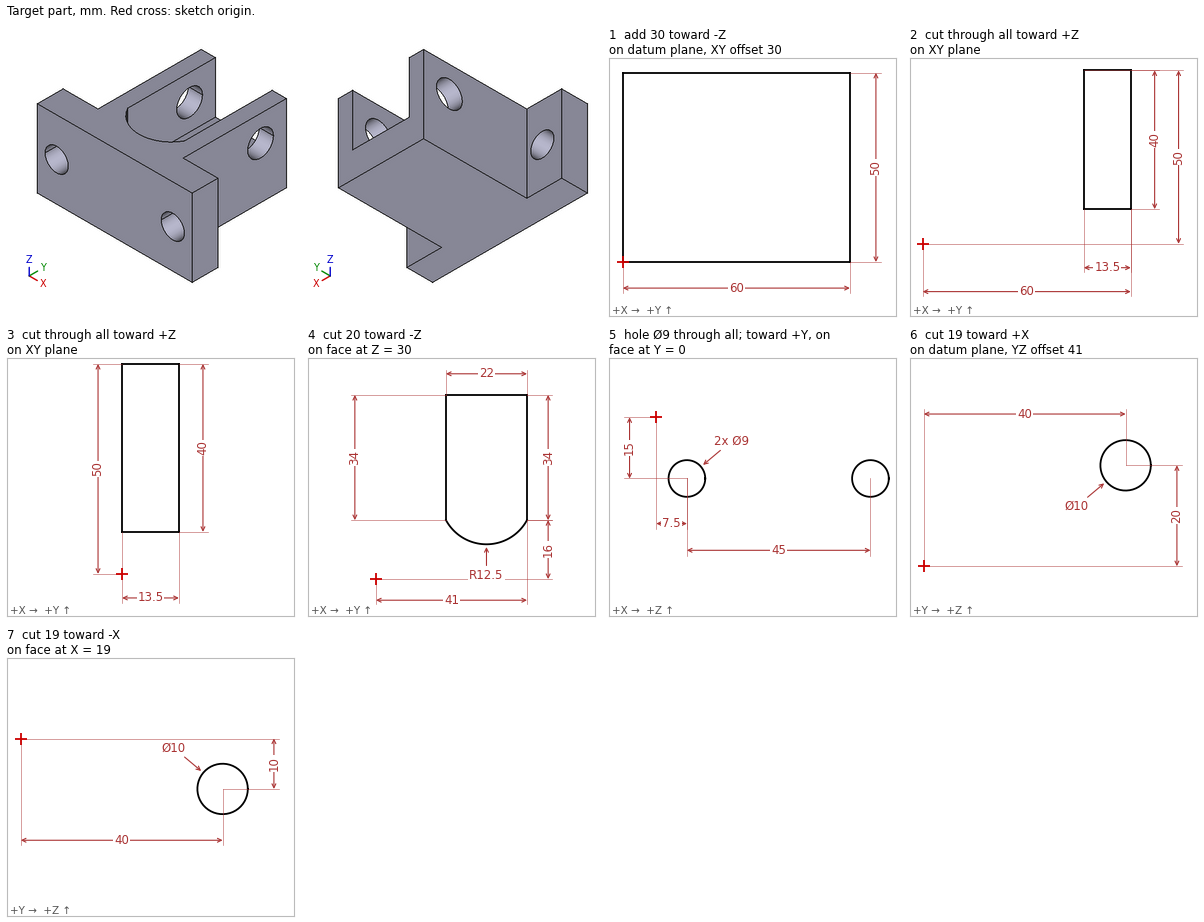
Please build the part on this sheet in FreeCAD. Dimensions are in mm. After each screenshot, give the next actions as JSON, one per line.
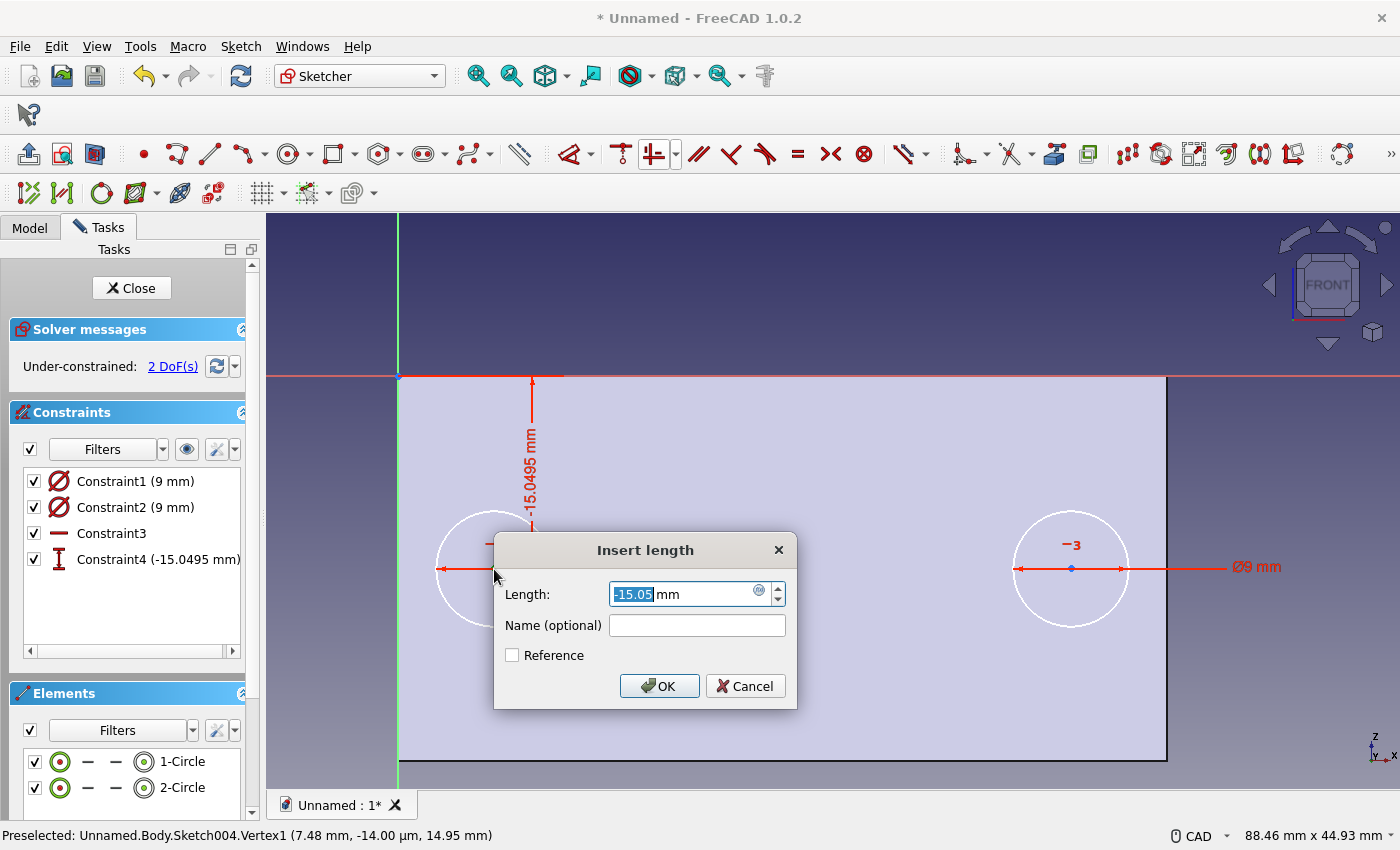
{"action": "type", "text": "-15"}
{"action": "key", "text": "Return"}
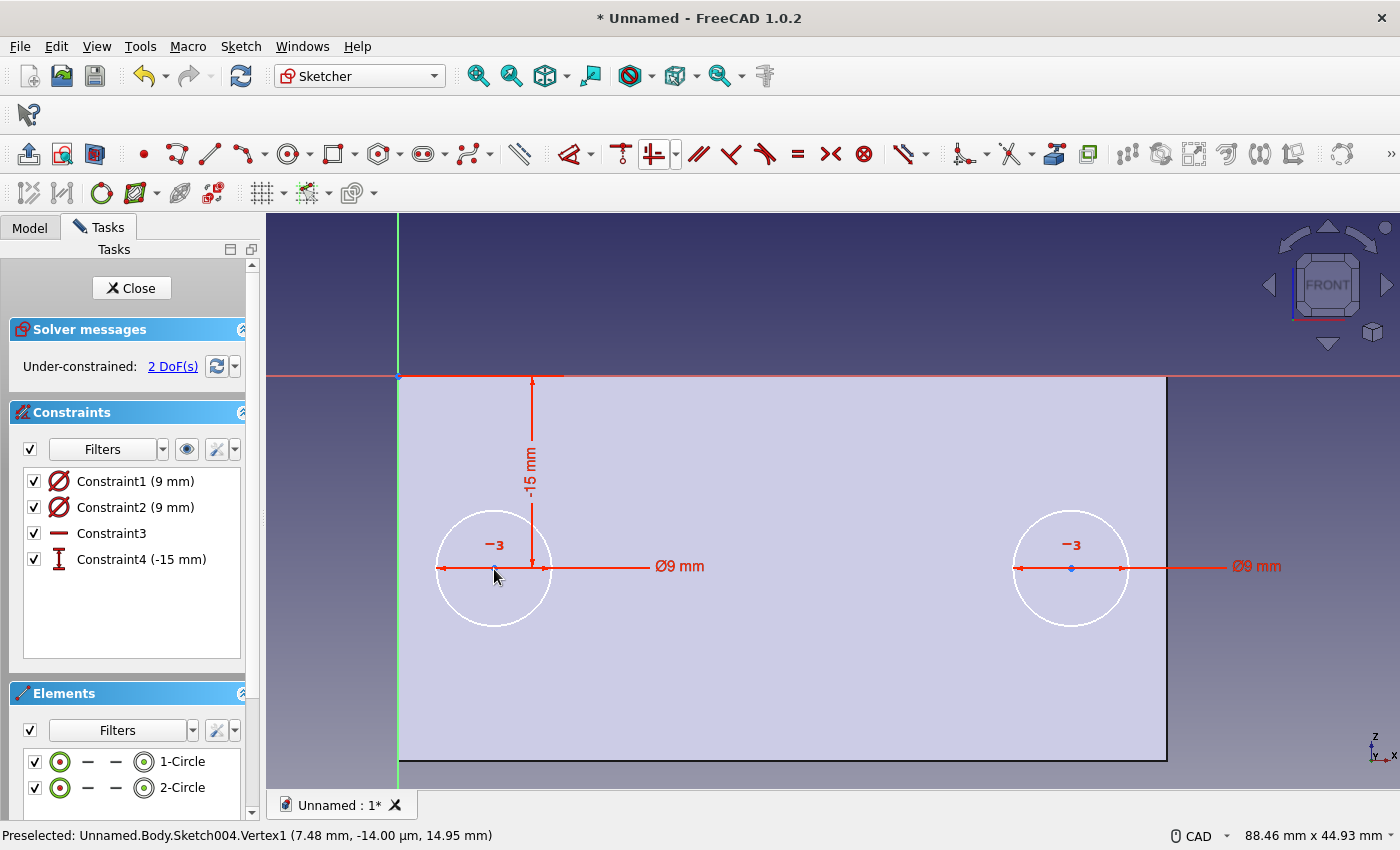
{"action": "left_click", "coordinate": [494, 568]}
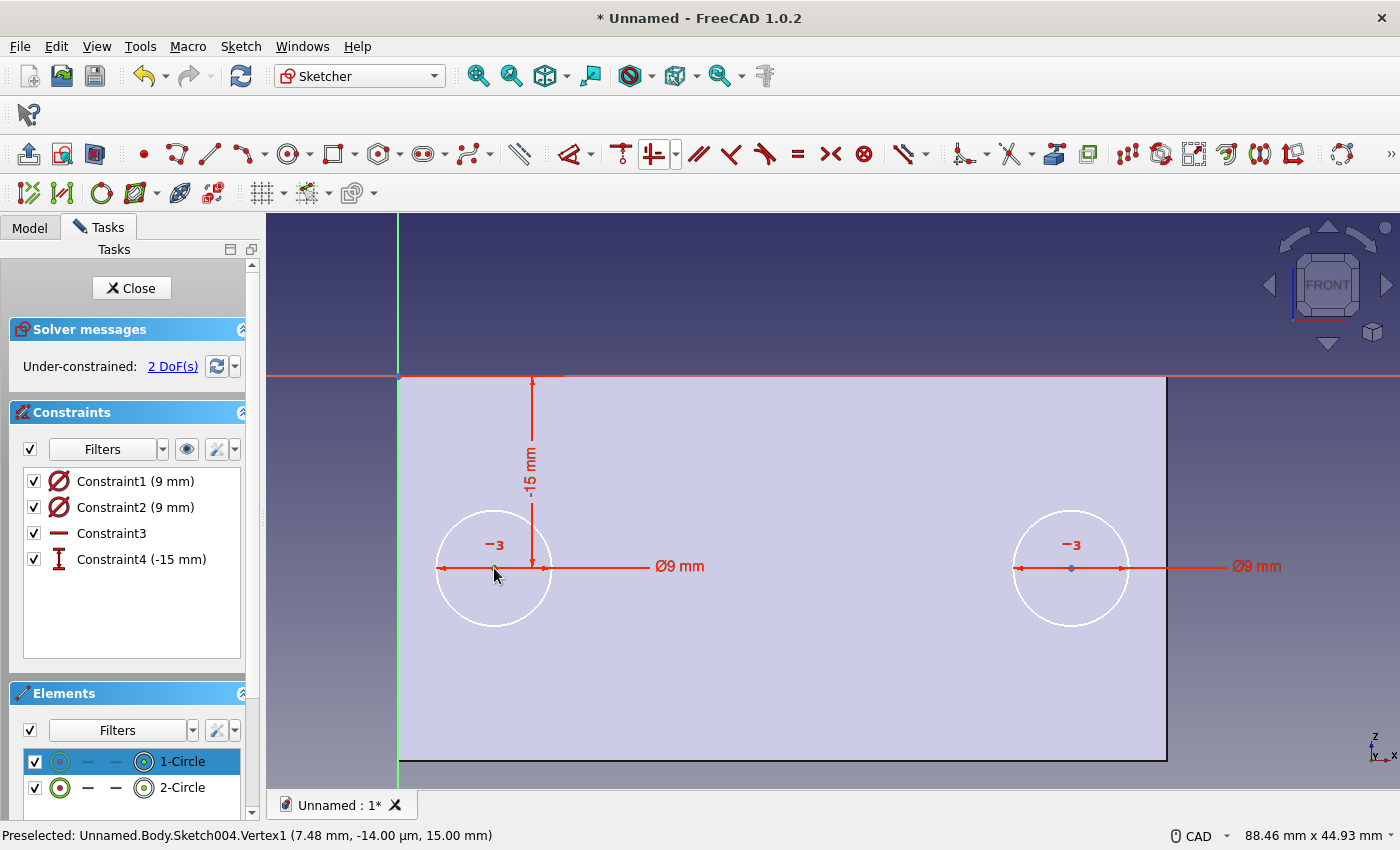
{"action": "key", "text": "l"}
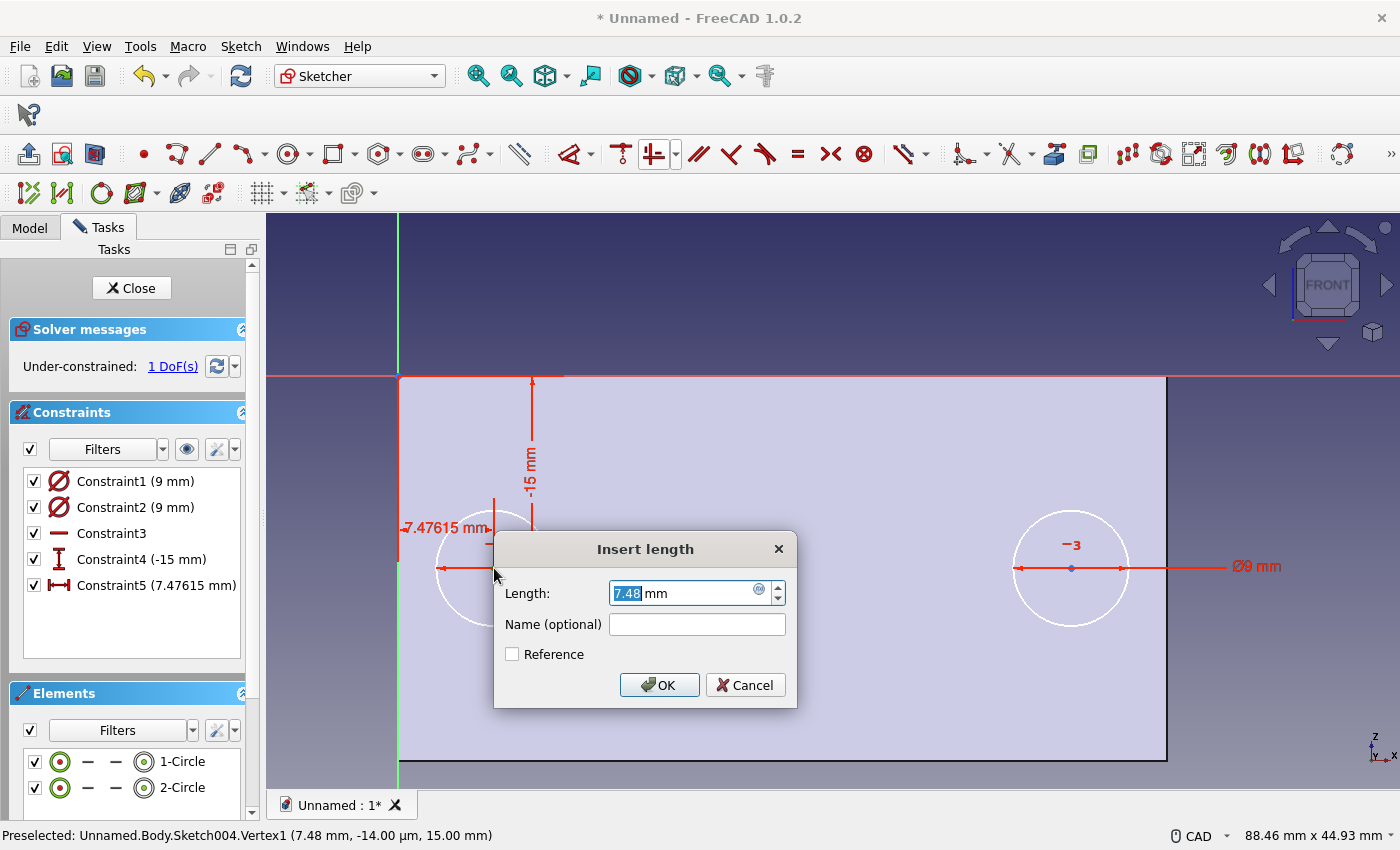
{"action": "type", "text": "7.5"}
{"action": "key", "text": "Return"}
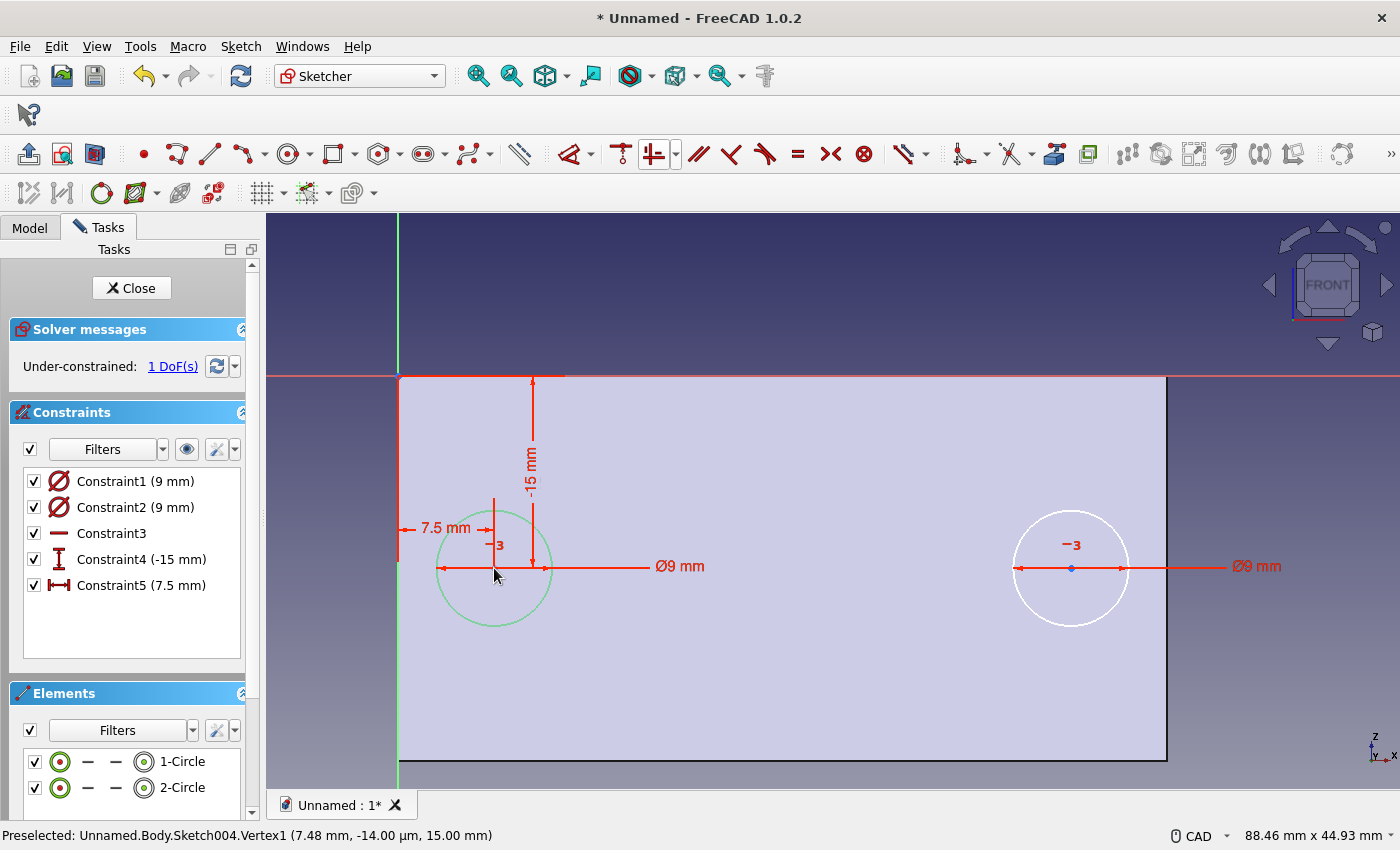
{"action": "left_click", "coordinate": [494, 568]}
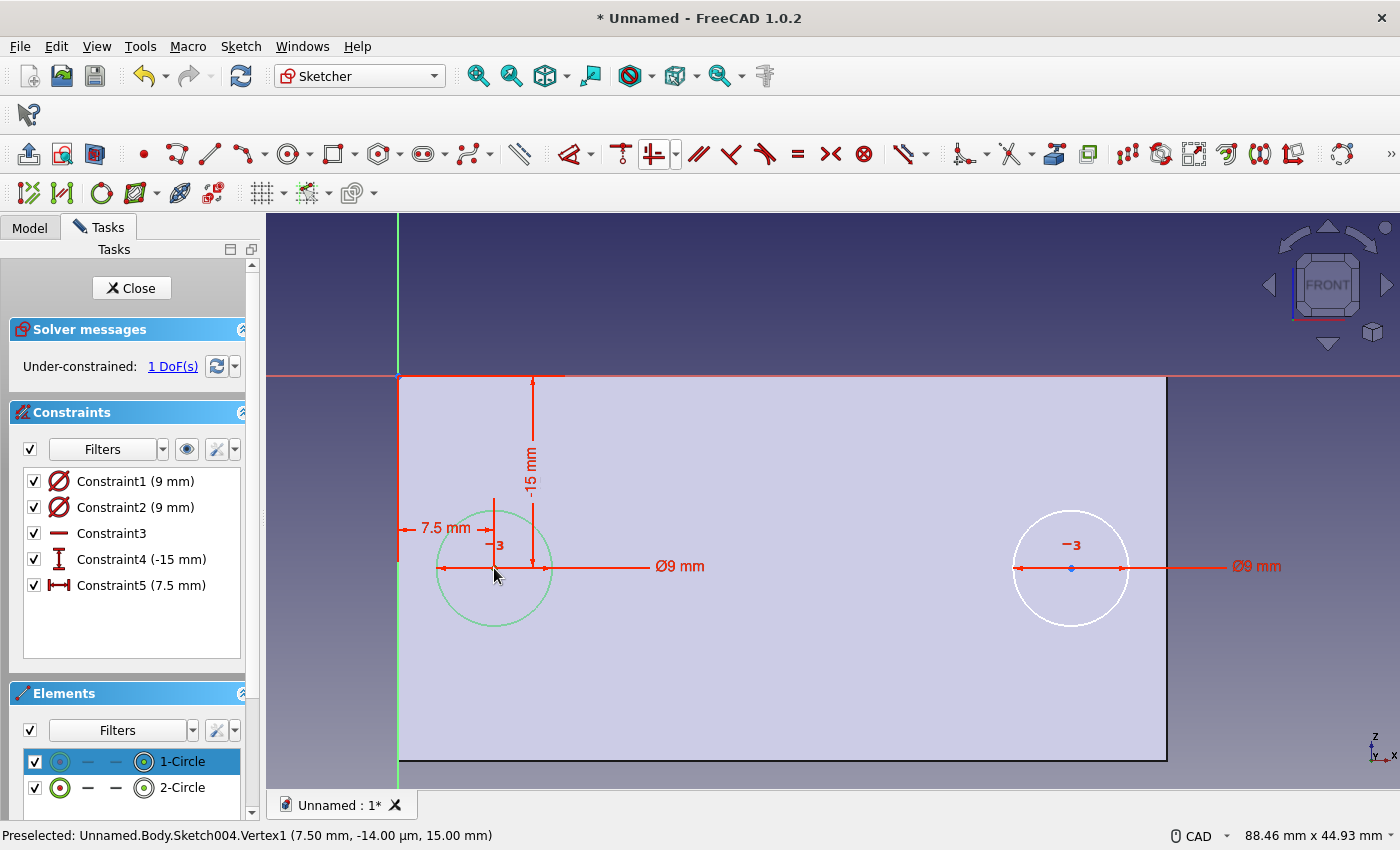
{"action": "left_click", "coordinate": [1071, 568]}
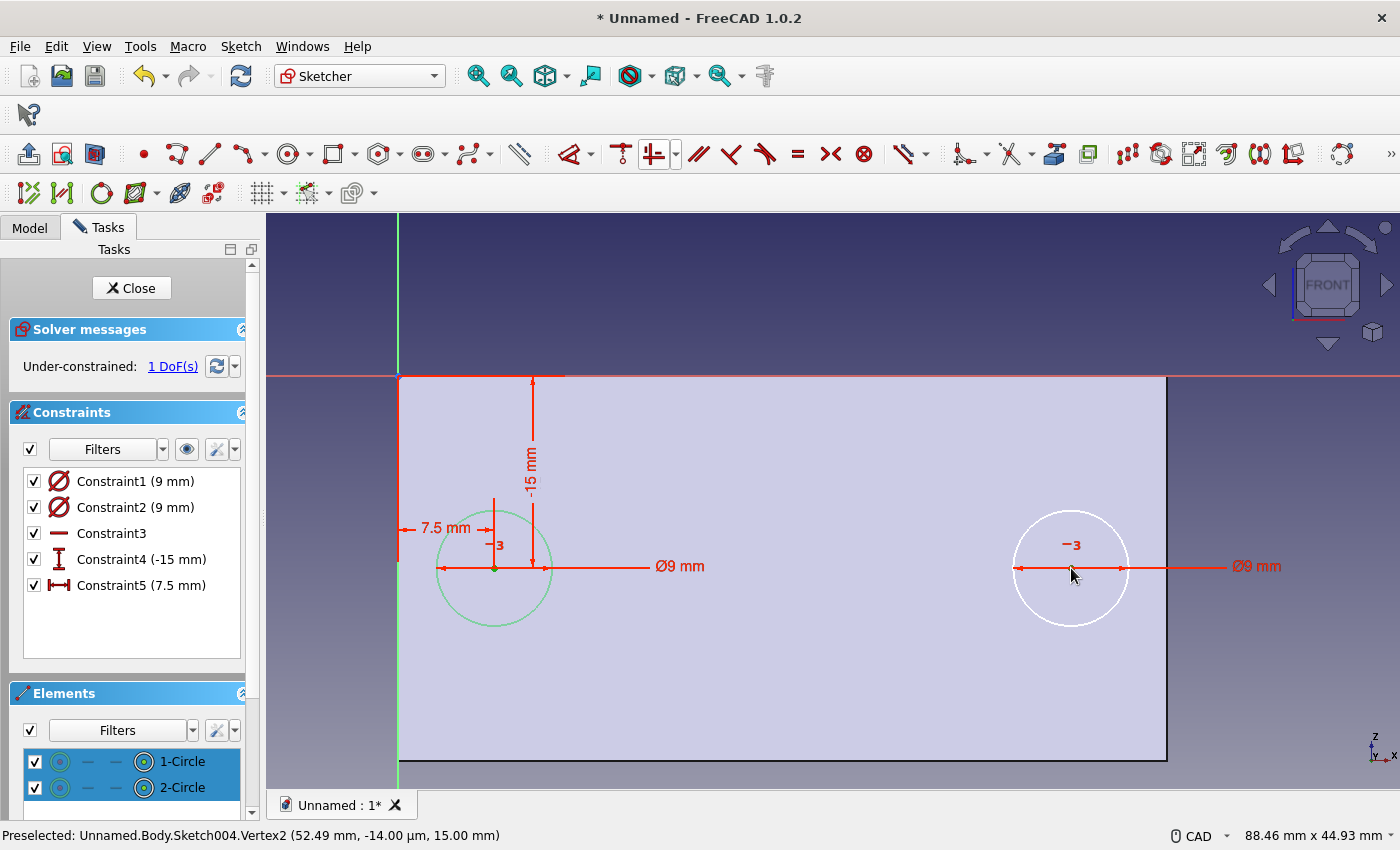
{"action": "key", "text": "l"}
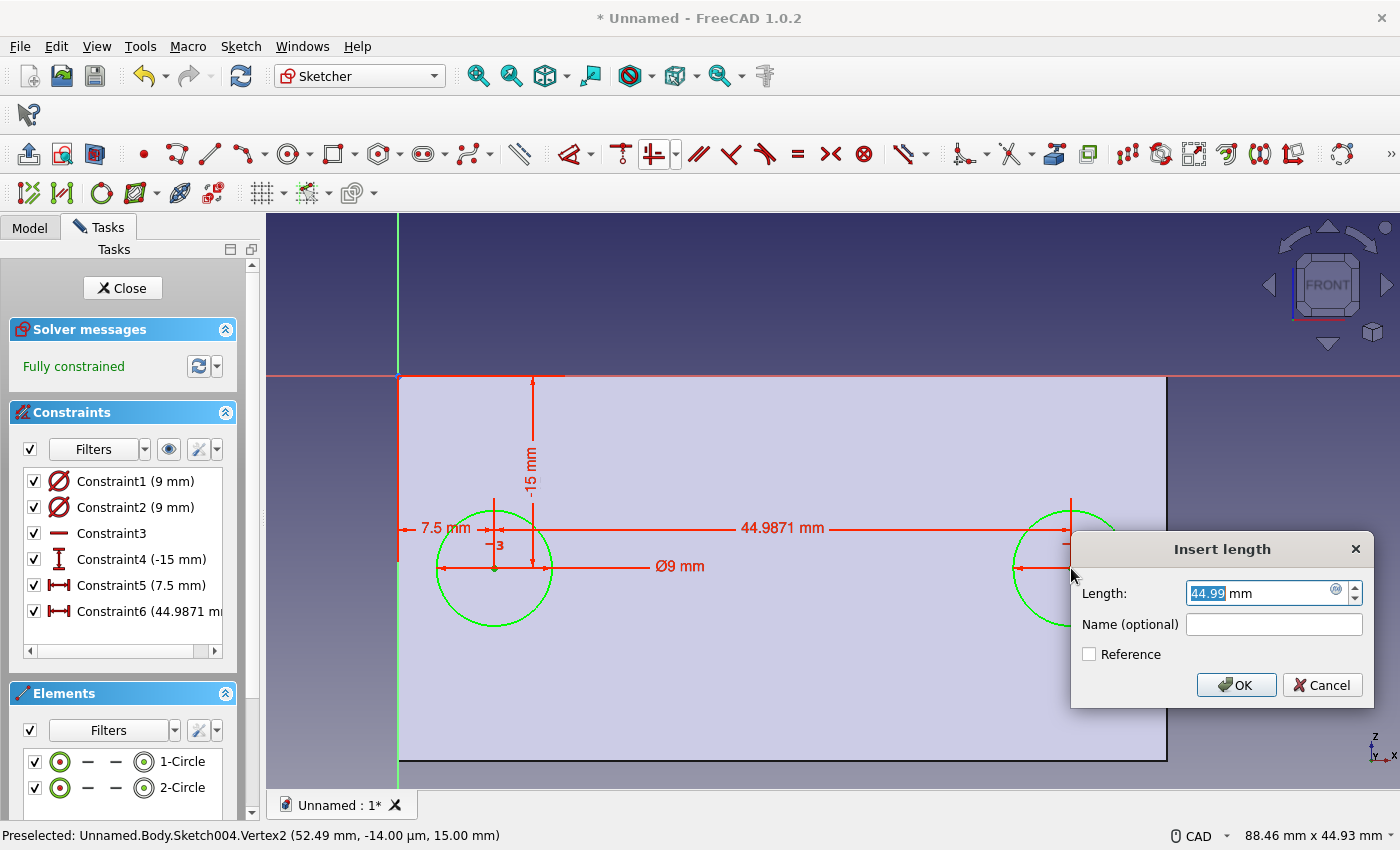
{"action": "type", "text": "45"}
{"action": "key", "text": "Return"}